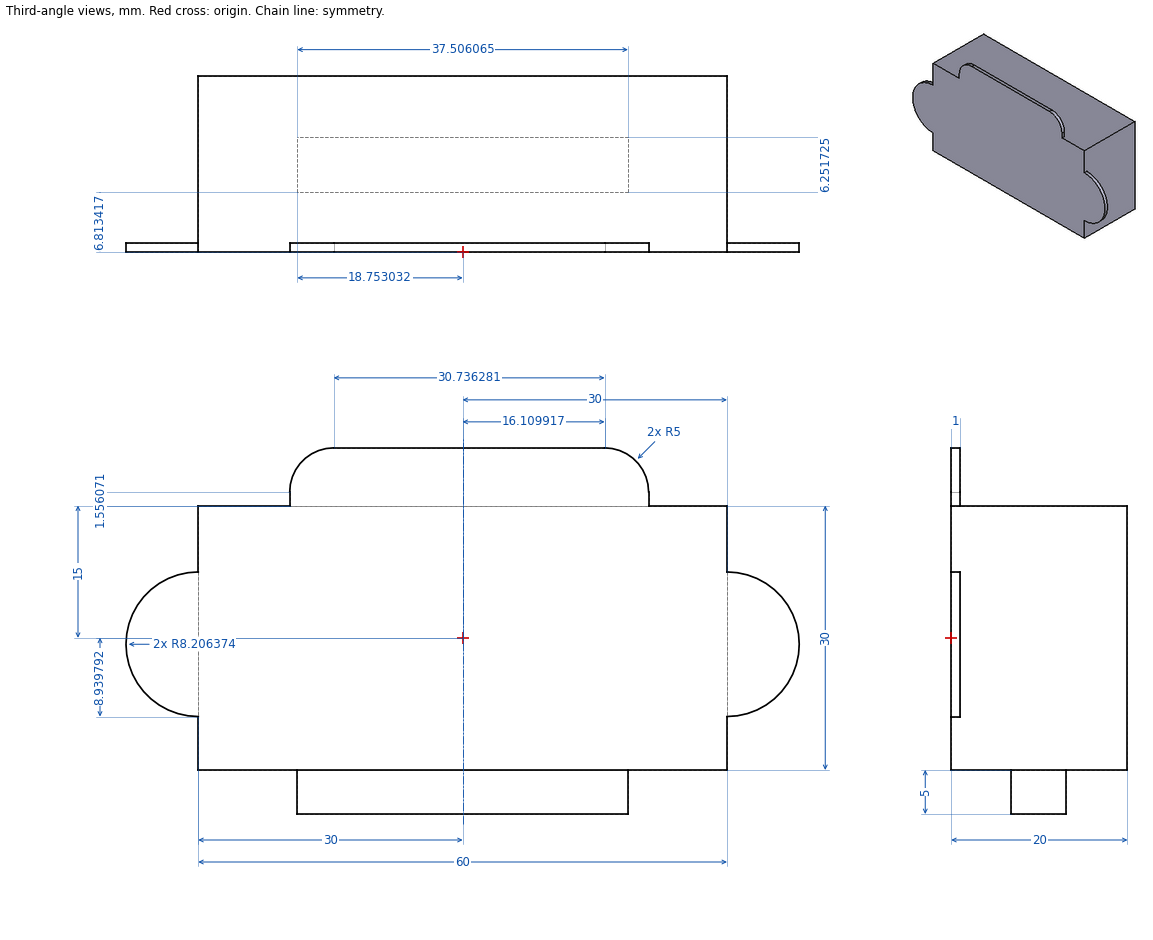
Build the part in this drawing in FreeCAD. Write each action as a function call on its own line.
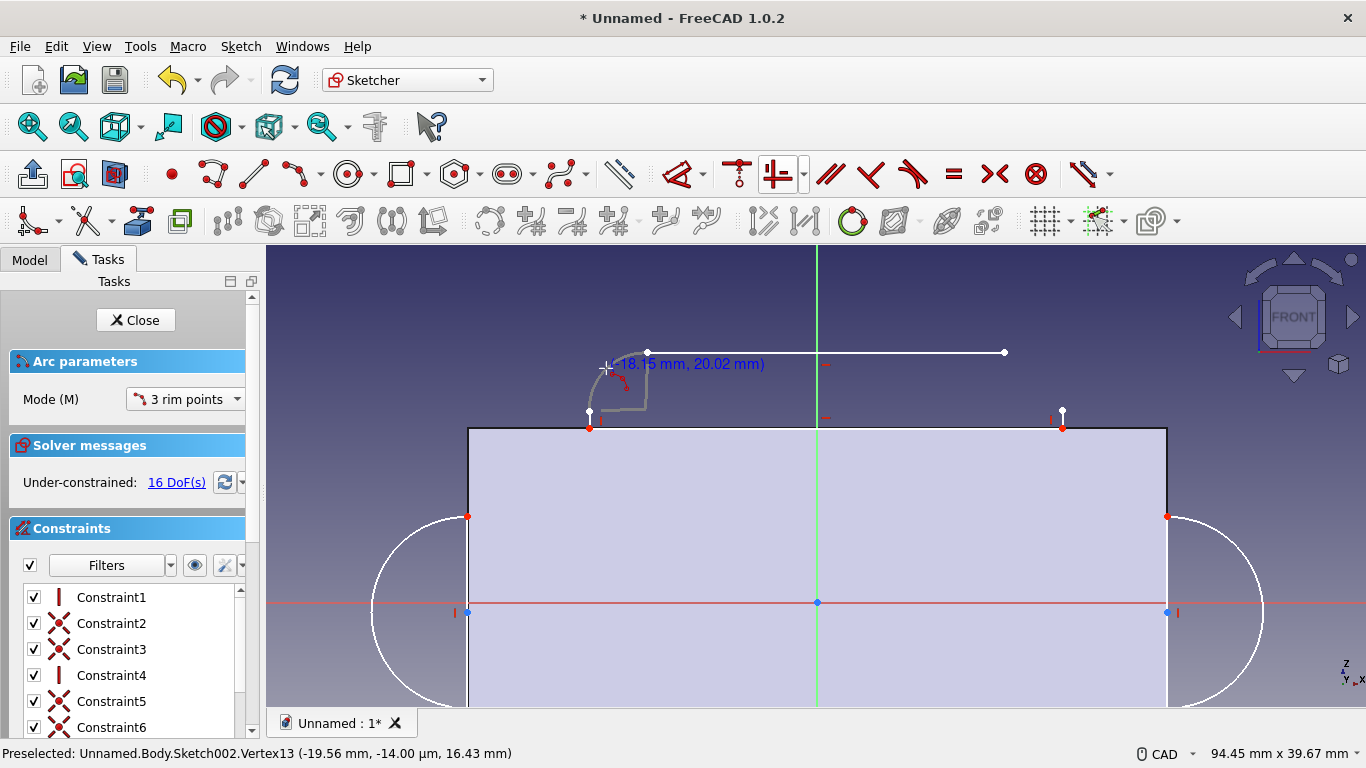
click(606, 369)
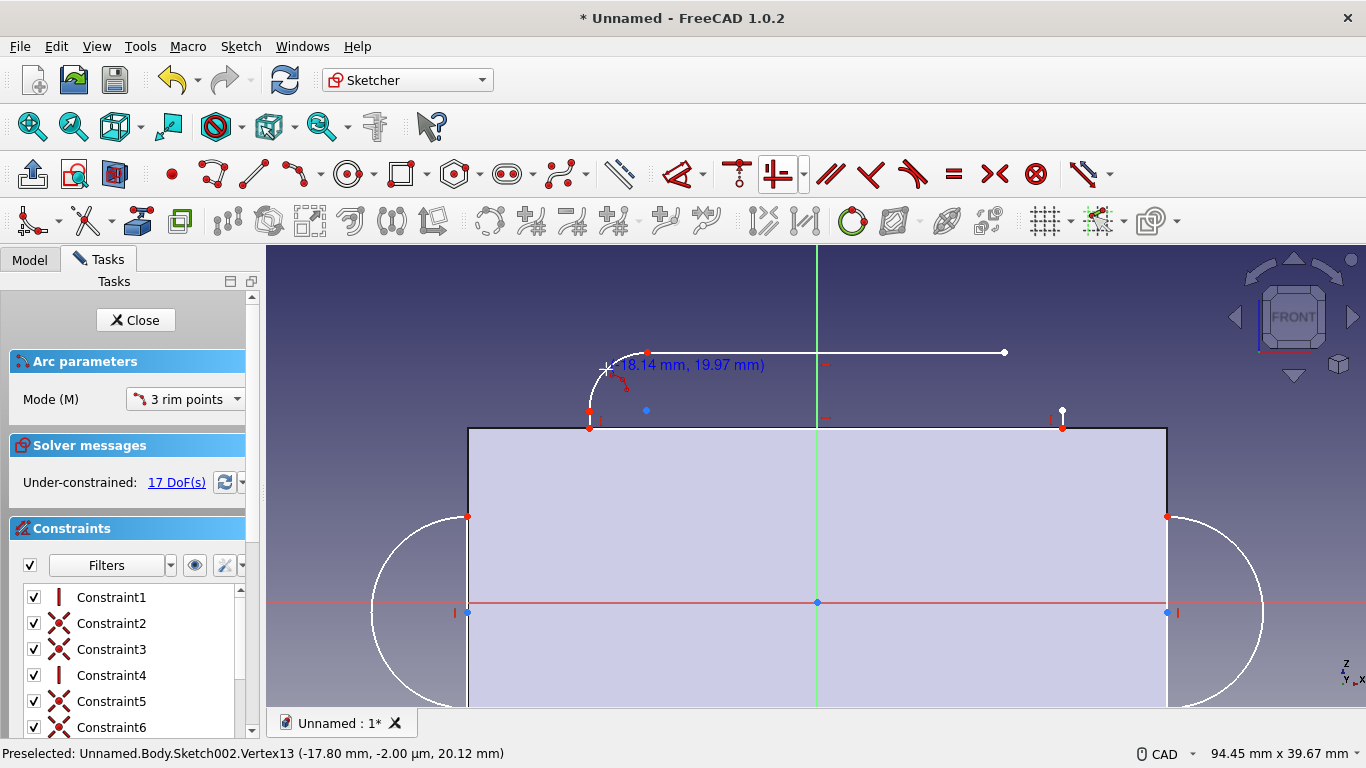
scroll(1063, 410, up, 3)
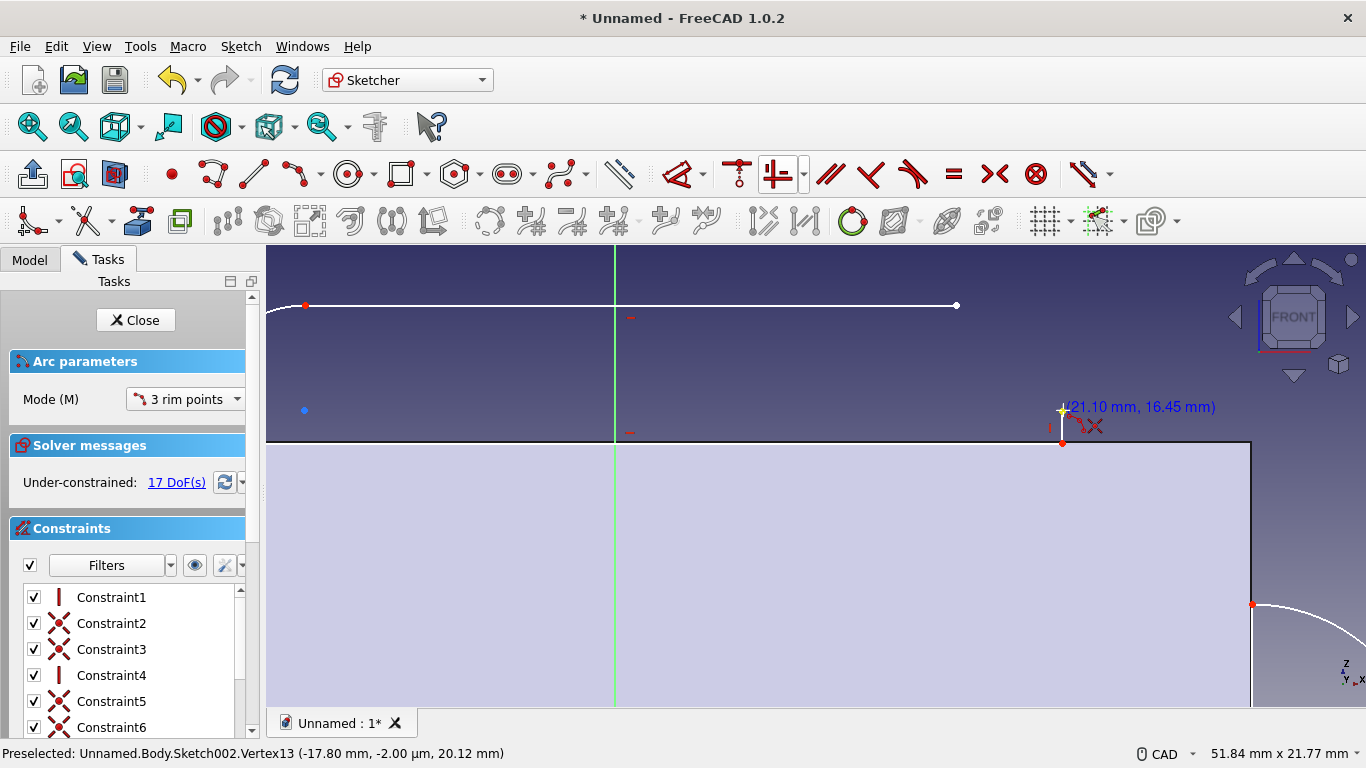
click(1062, 411)
click(957, 306)
click(1032, 334)
key(Escape)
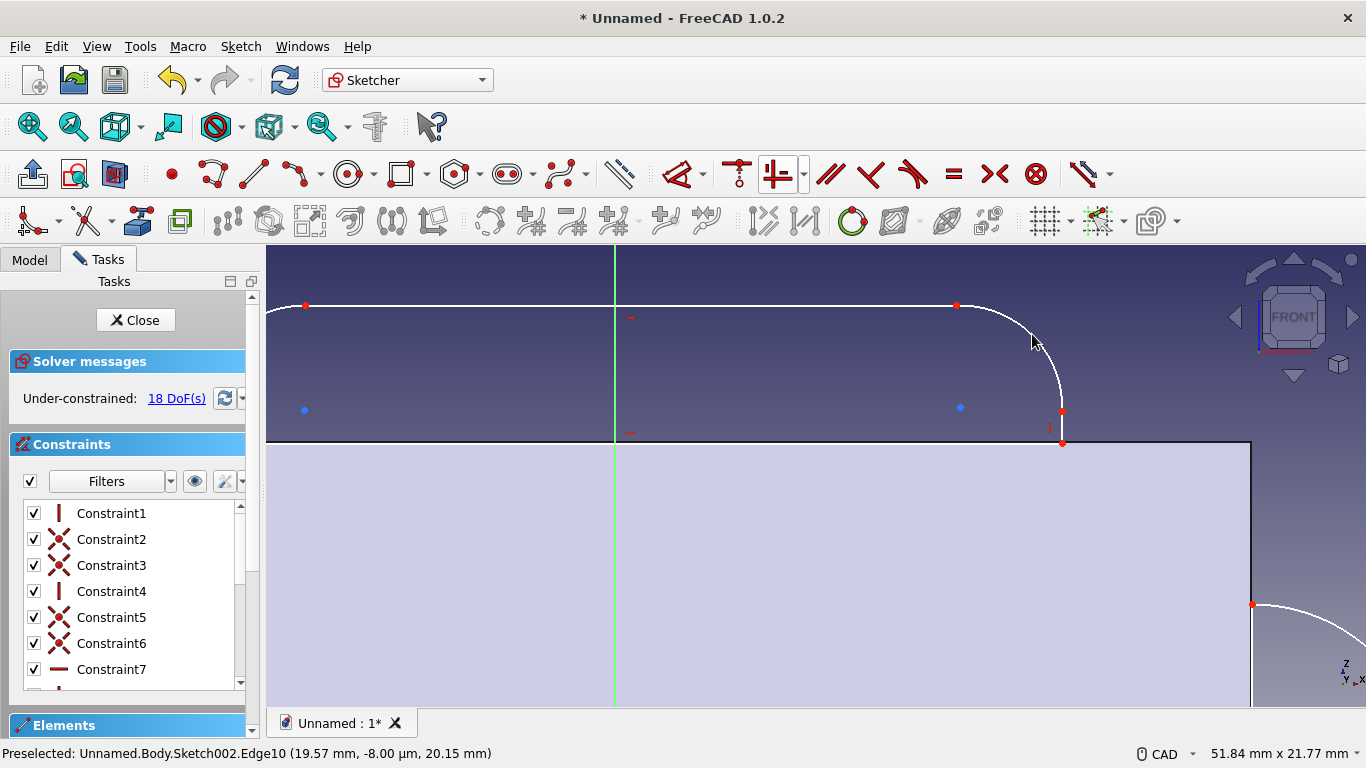
click(761, 306)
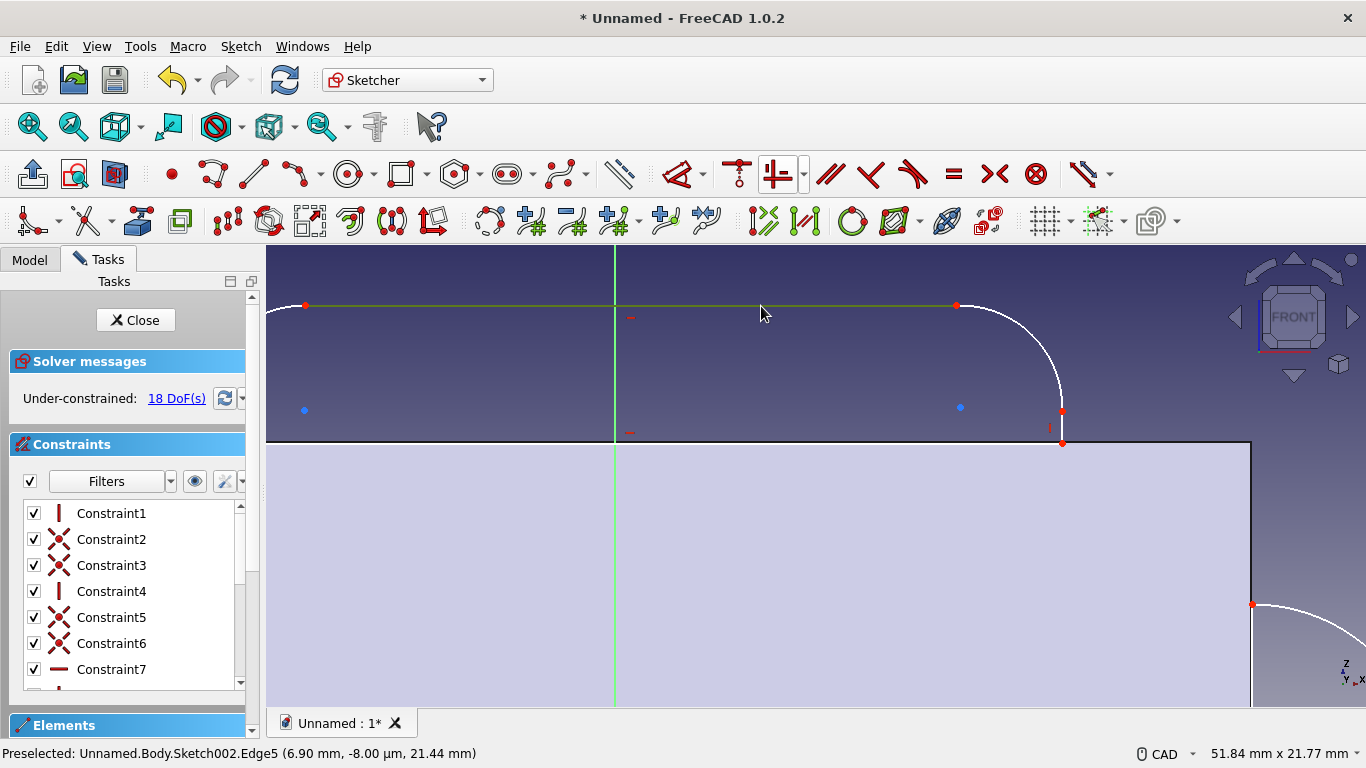
scroll(825, 388, down, 5)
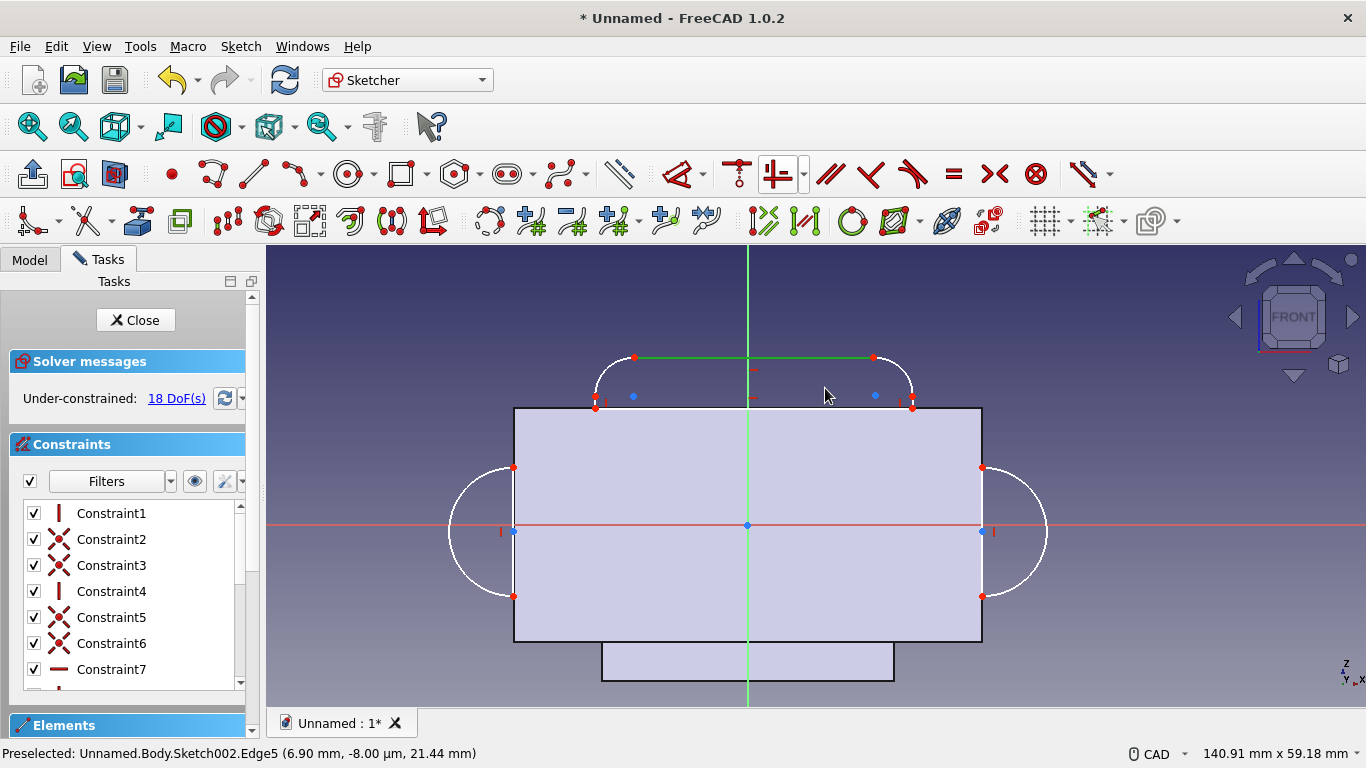
click(616, 362)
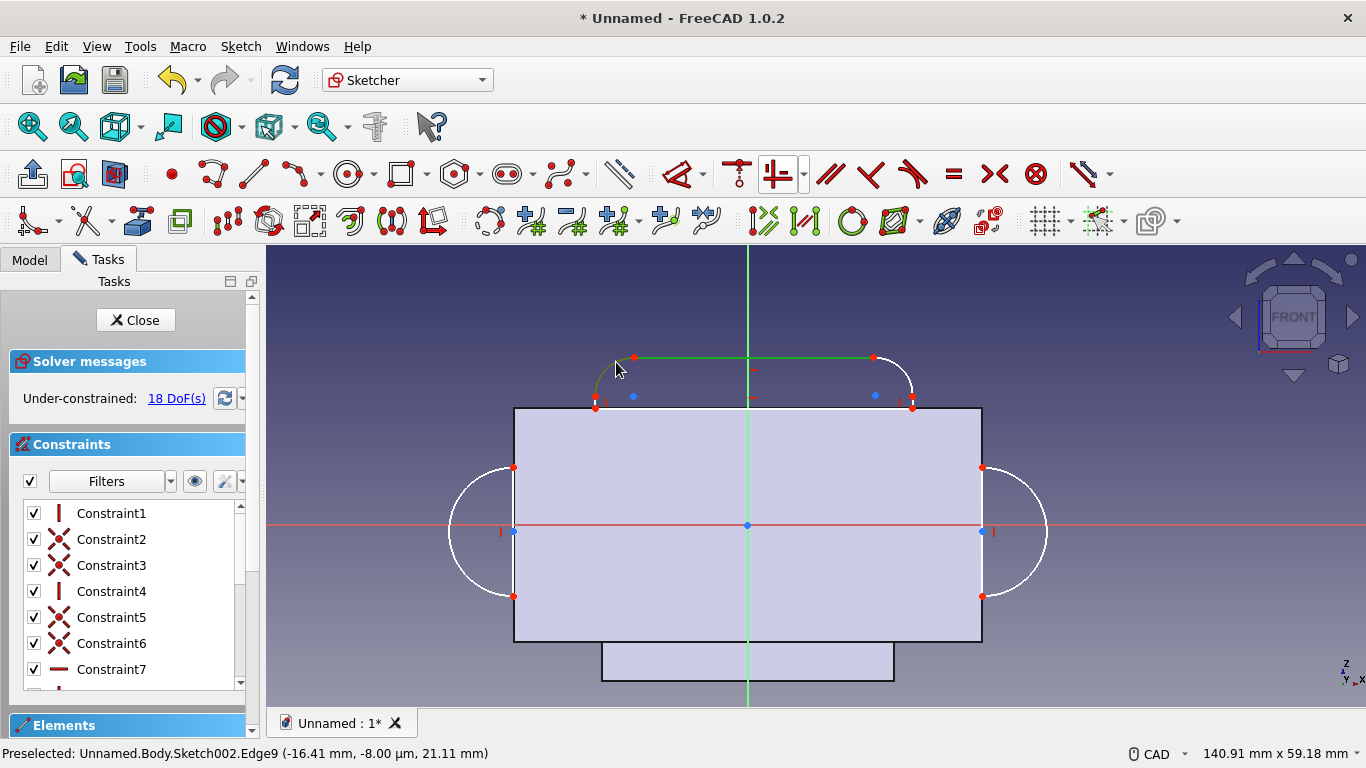
key(t)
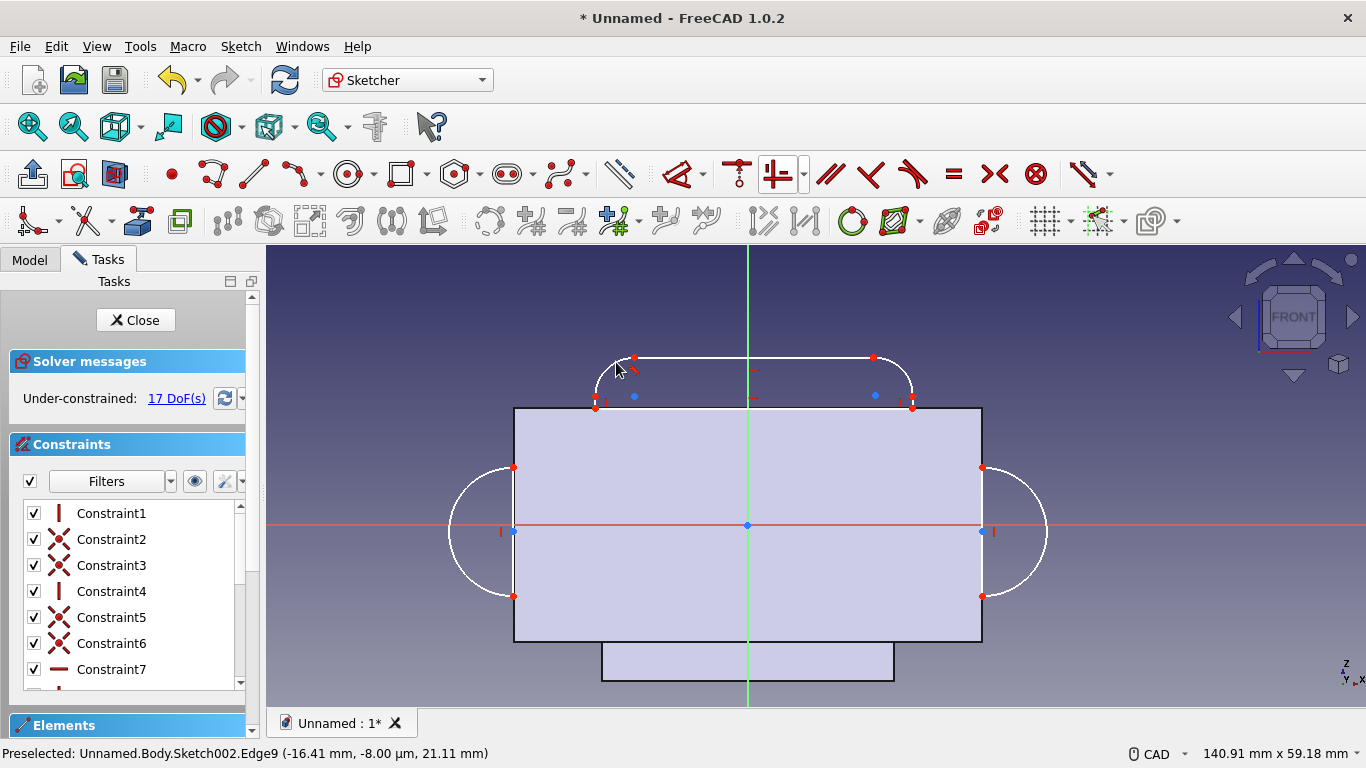
click(802, 358)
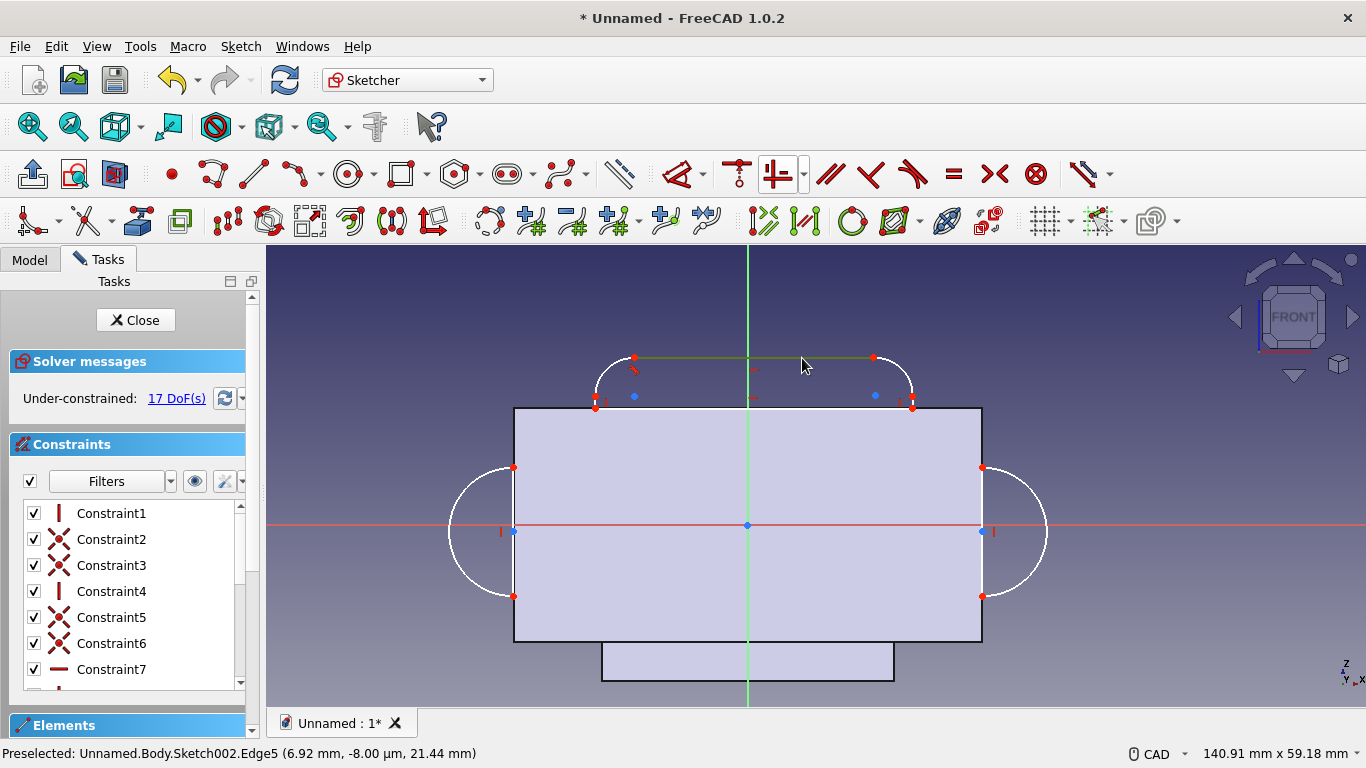
click(909, 379)